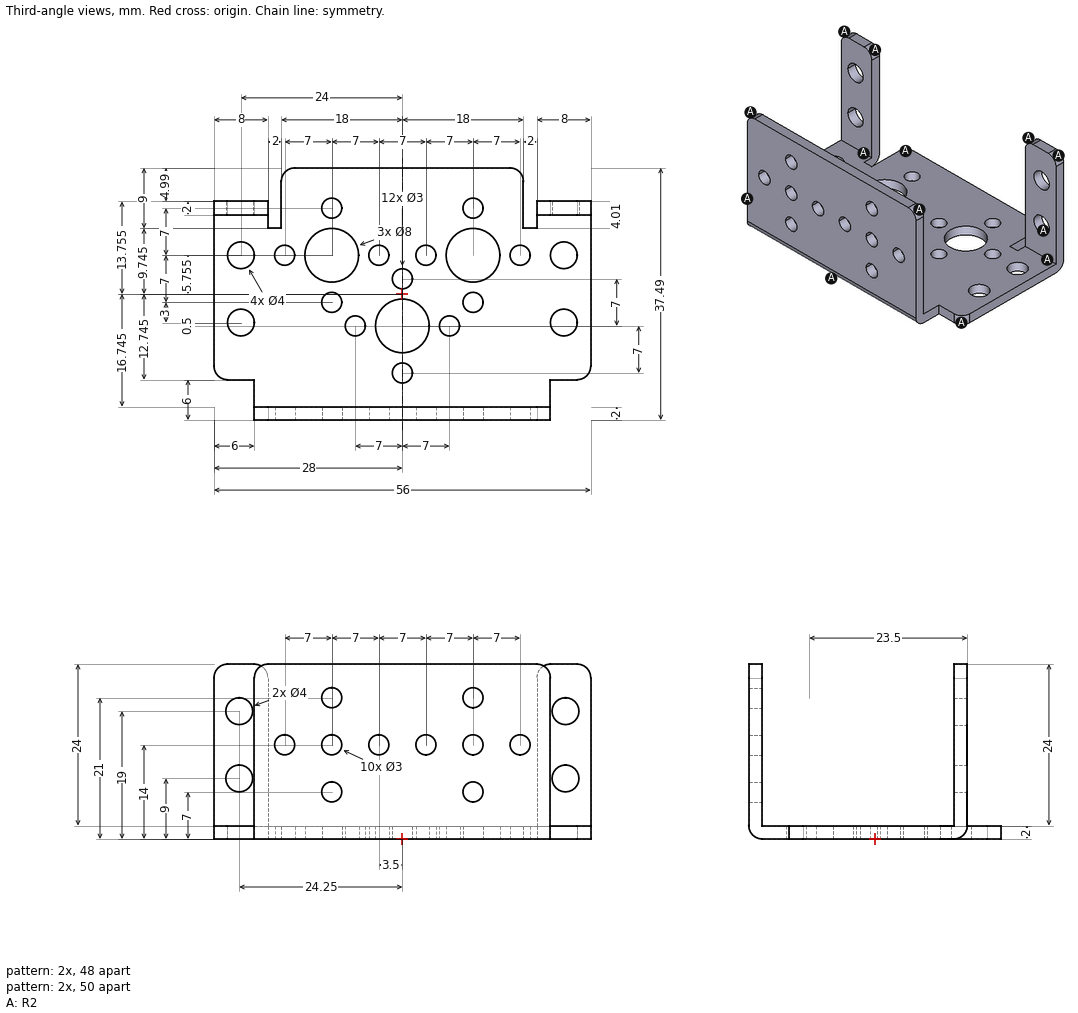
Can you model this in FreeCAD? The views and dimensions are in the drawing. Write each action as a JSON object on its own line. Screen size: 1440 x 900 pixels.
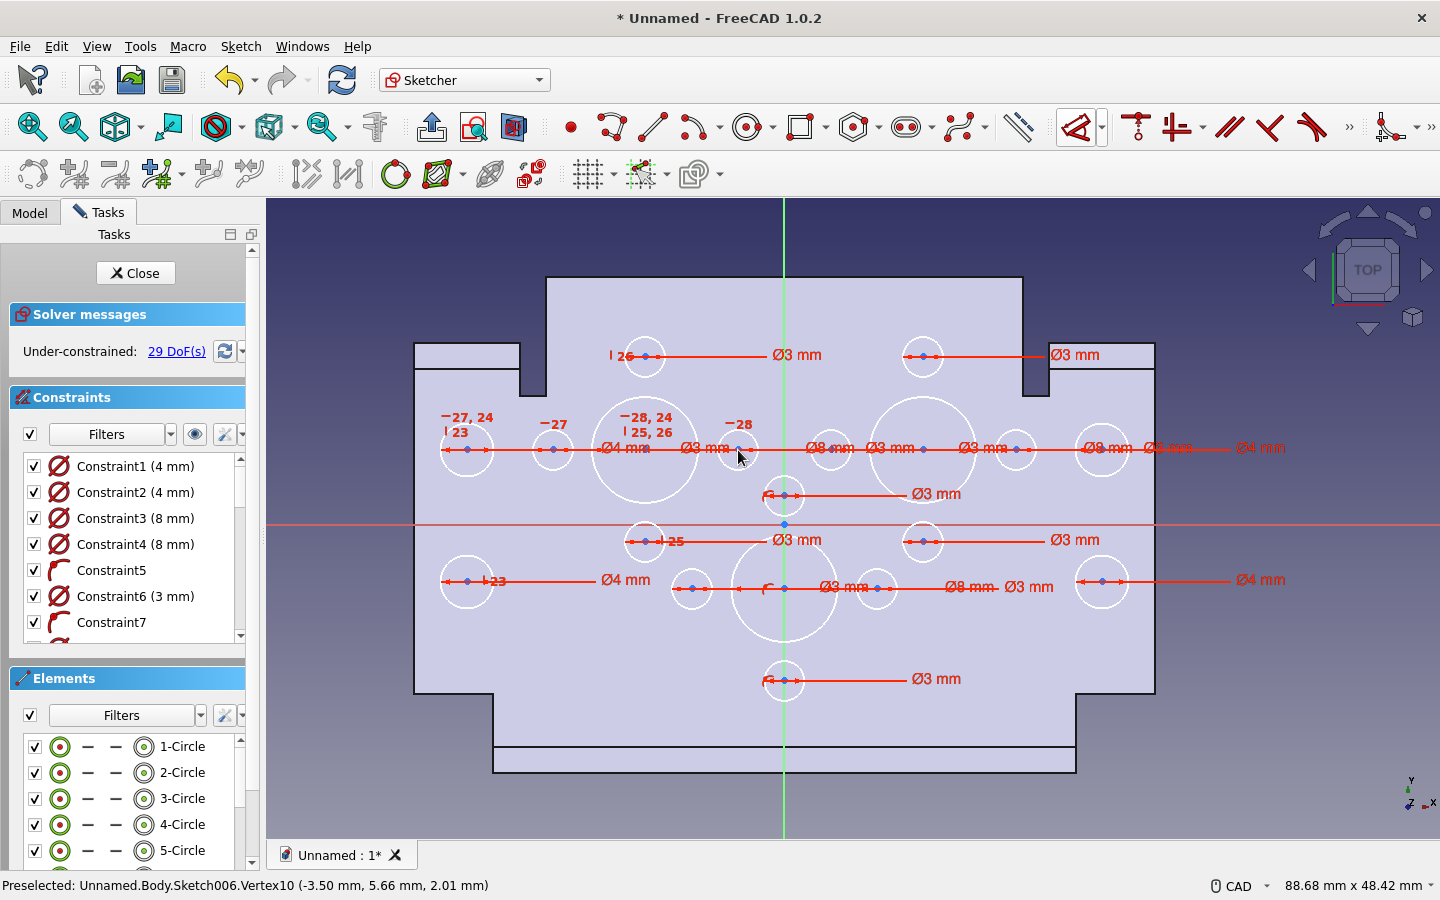
{"action": "left_click", "coordinate": [784, 589]}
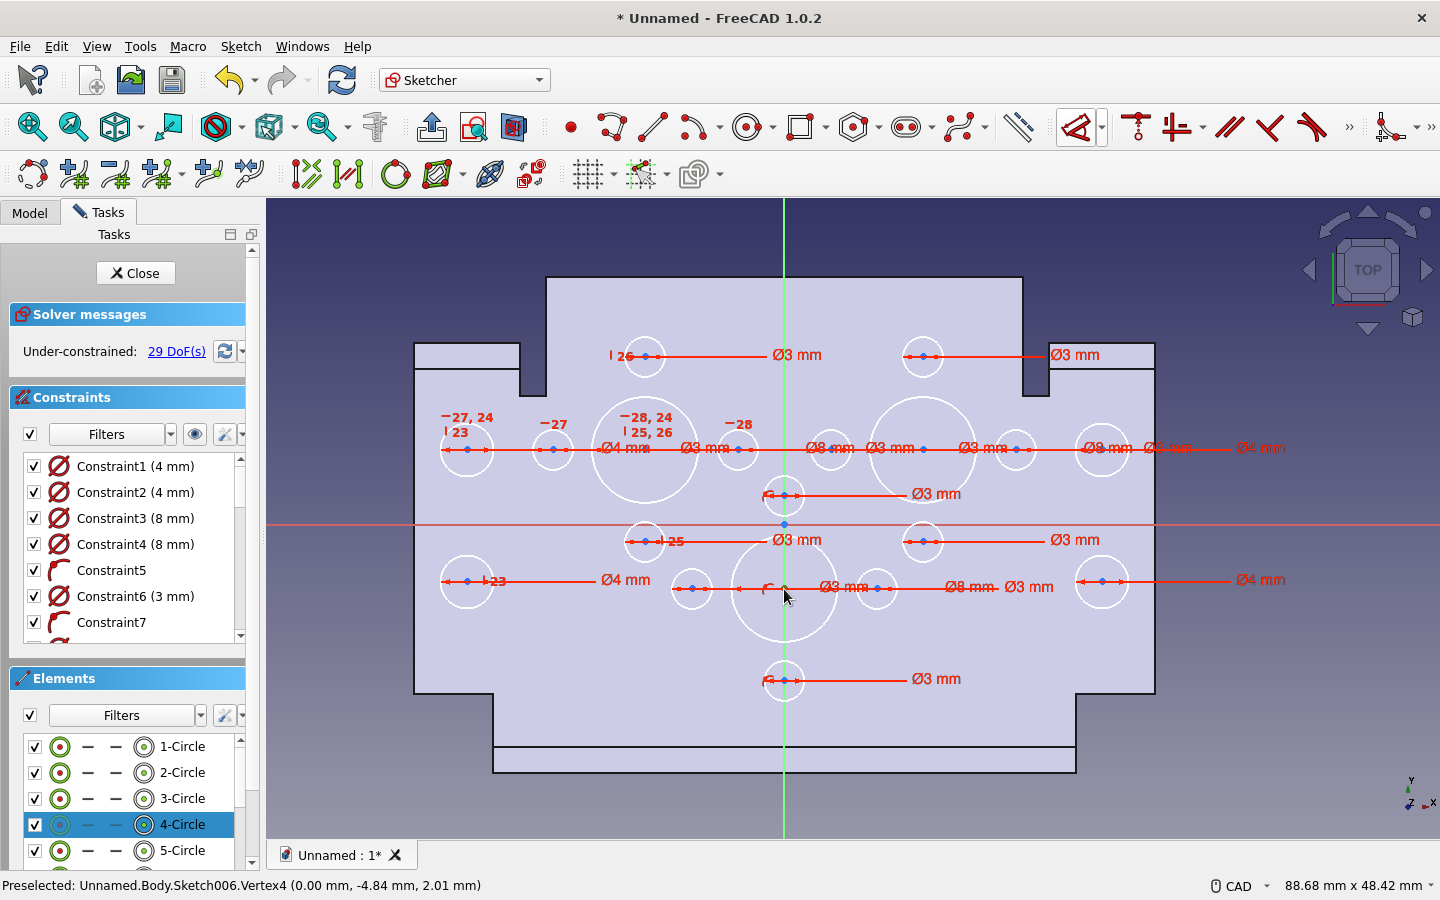
{"action": "left_click", "coordinate": [692, 589]}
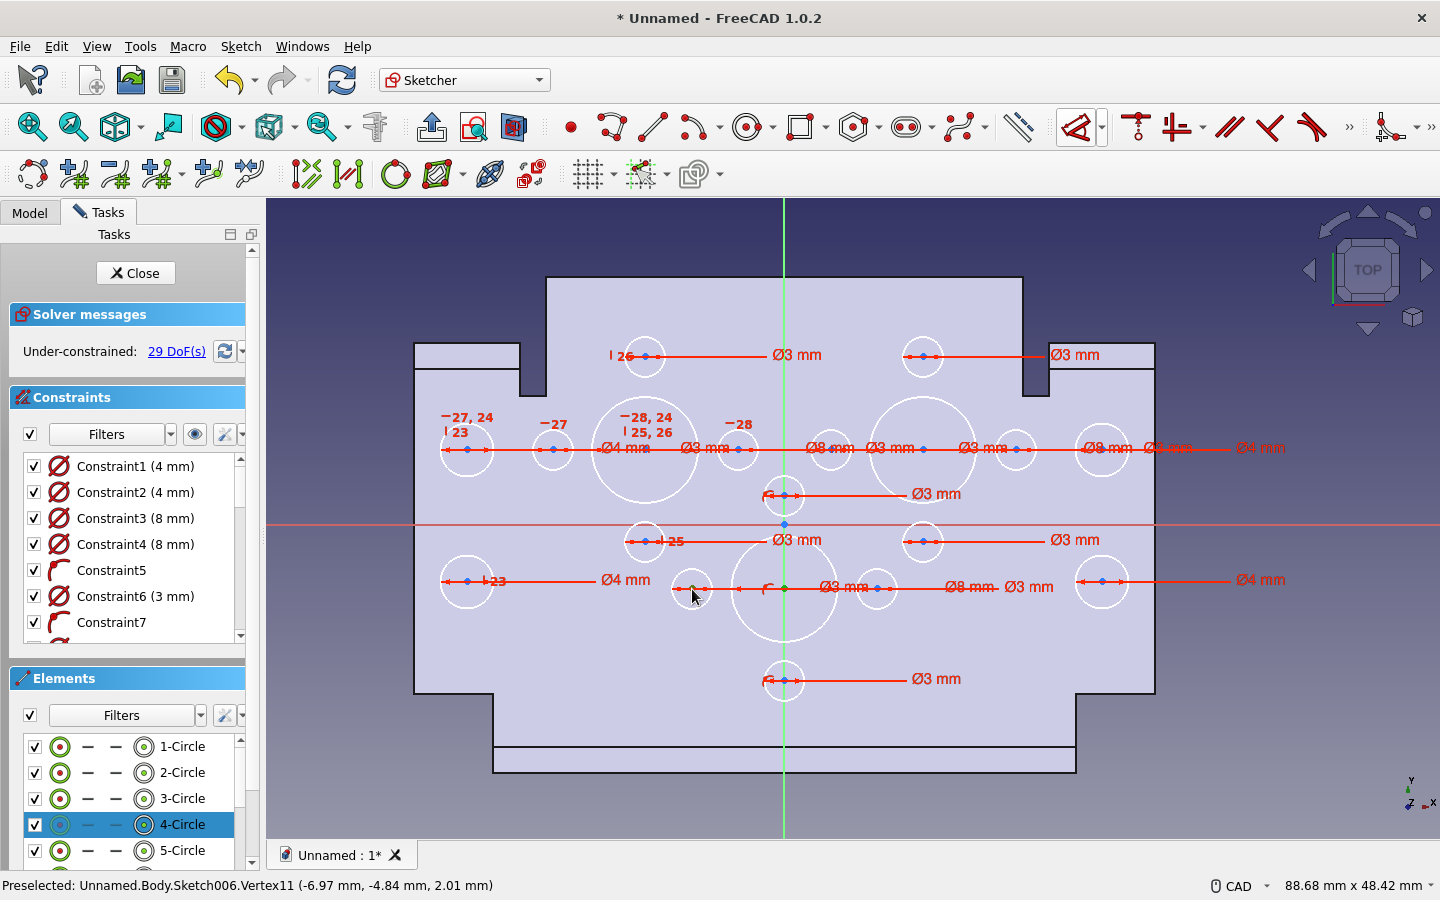
{"action": "key", "text": "h"}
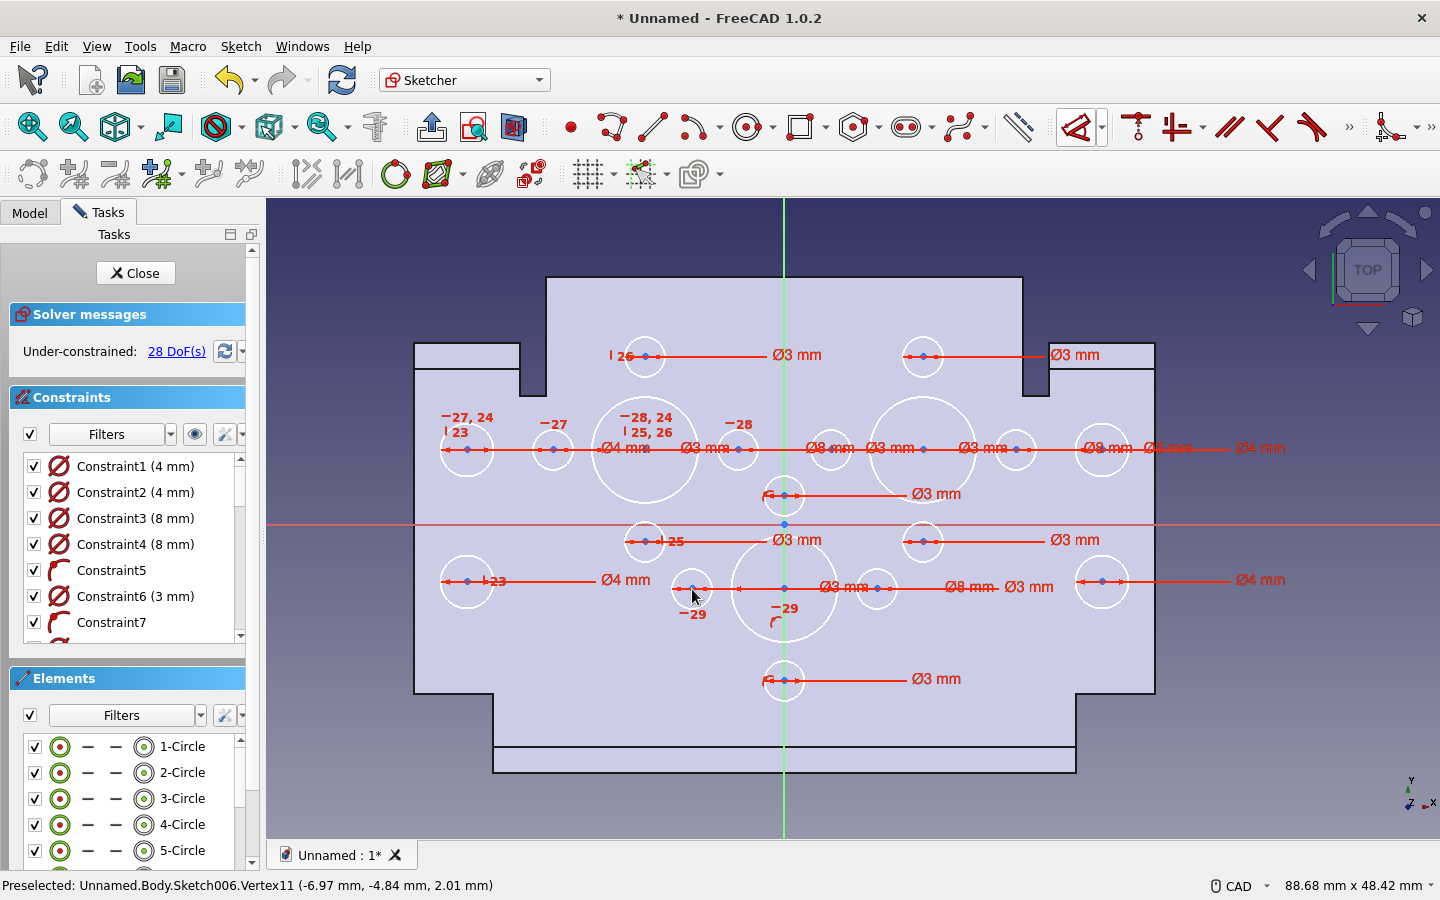
{"action": "left_click", "coordinate": [784, 589]}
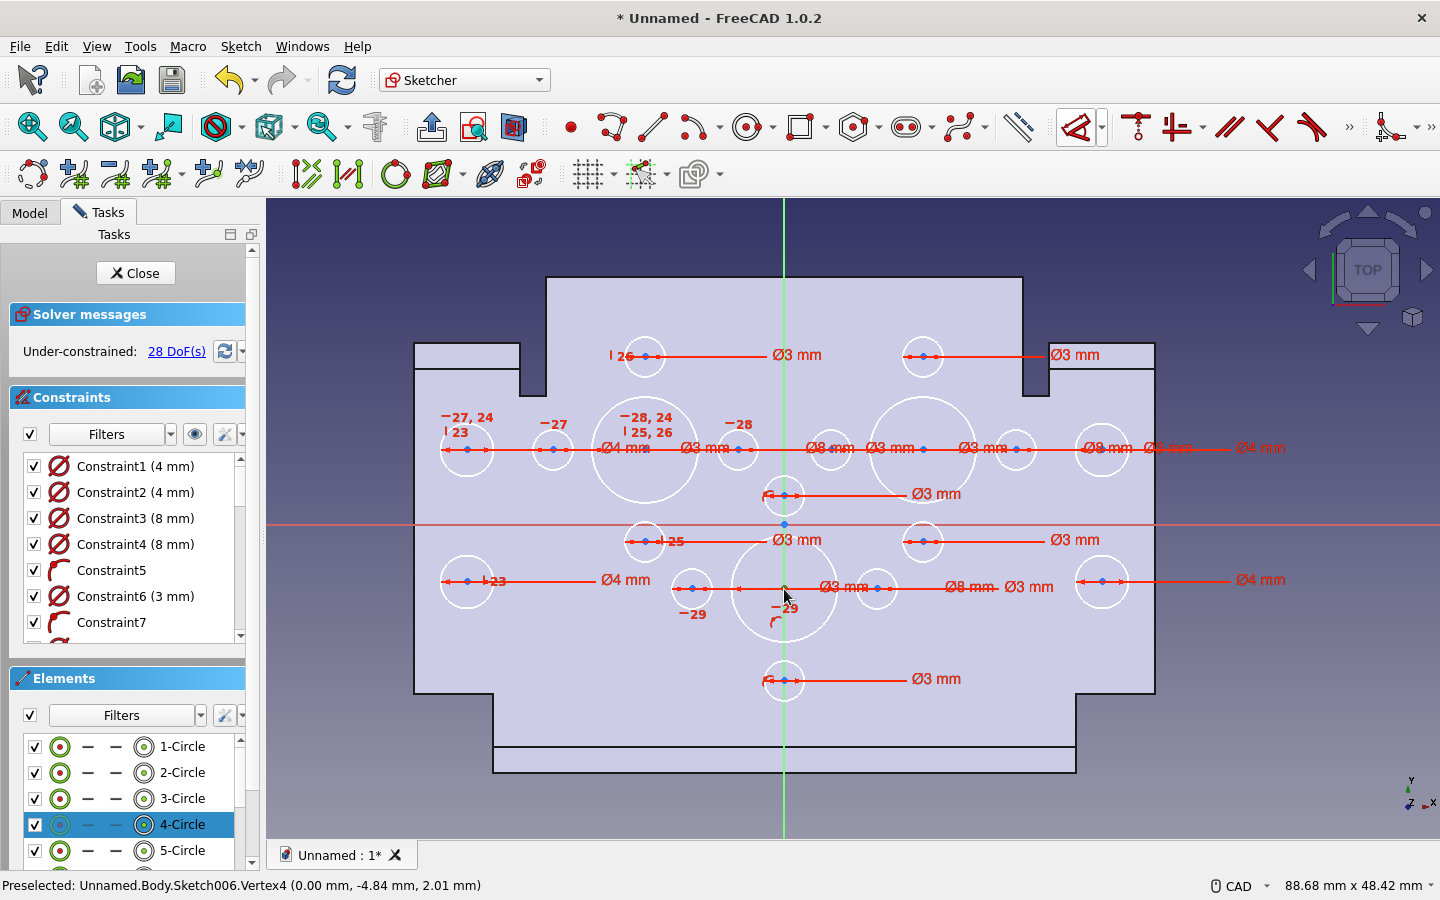
{"action": "left_click", "coordinate": [877, 589]}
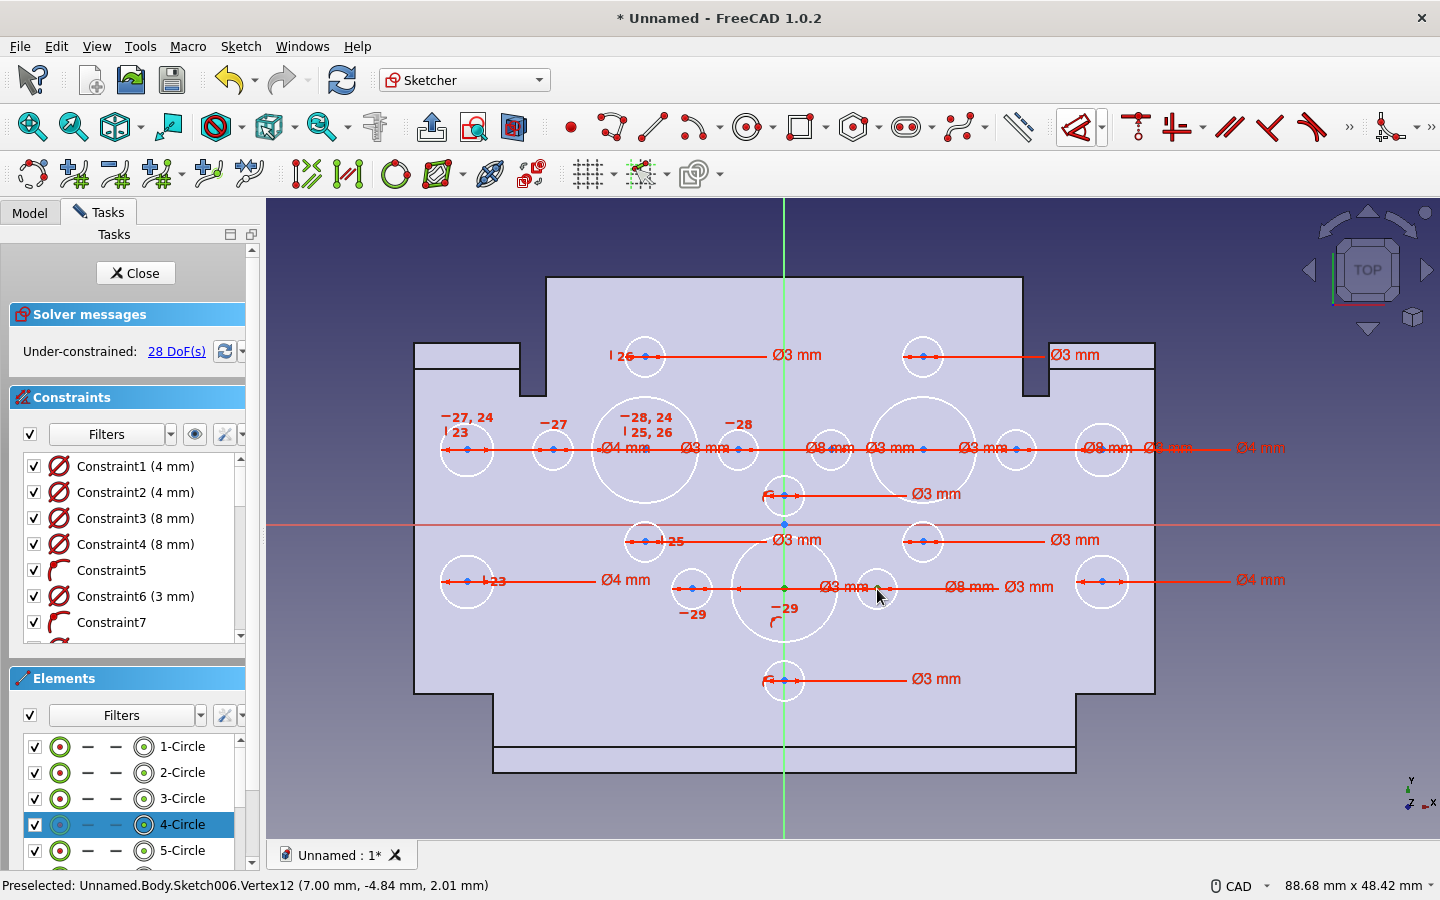
{"action": "key", "text": "h"}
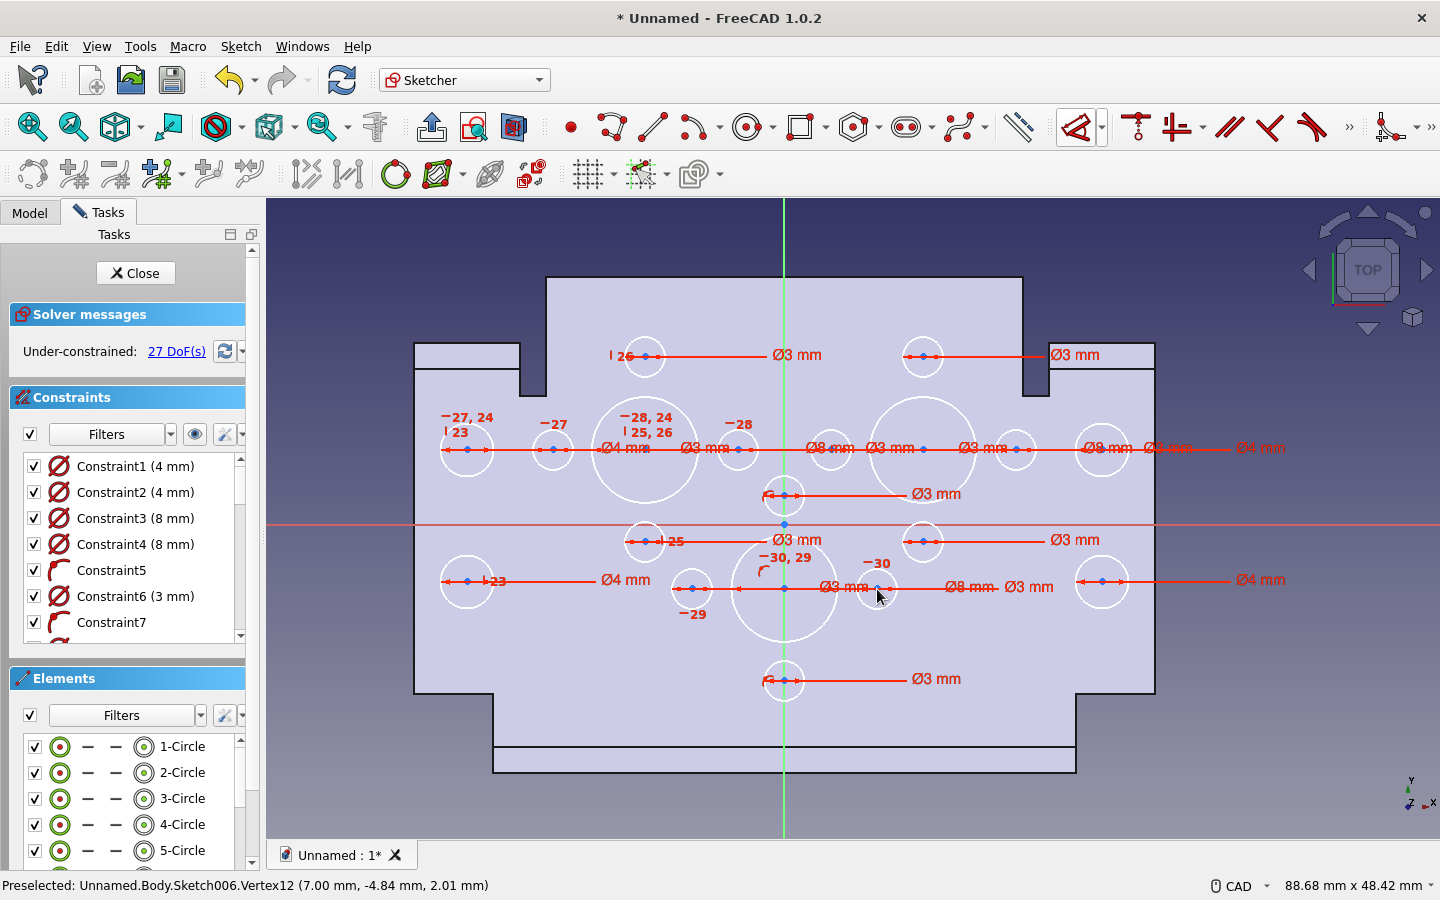
{"action": "left_click", "coordinate": [645, 357]}